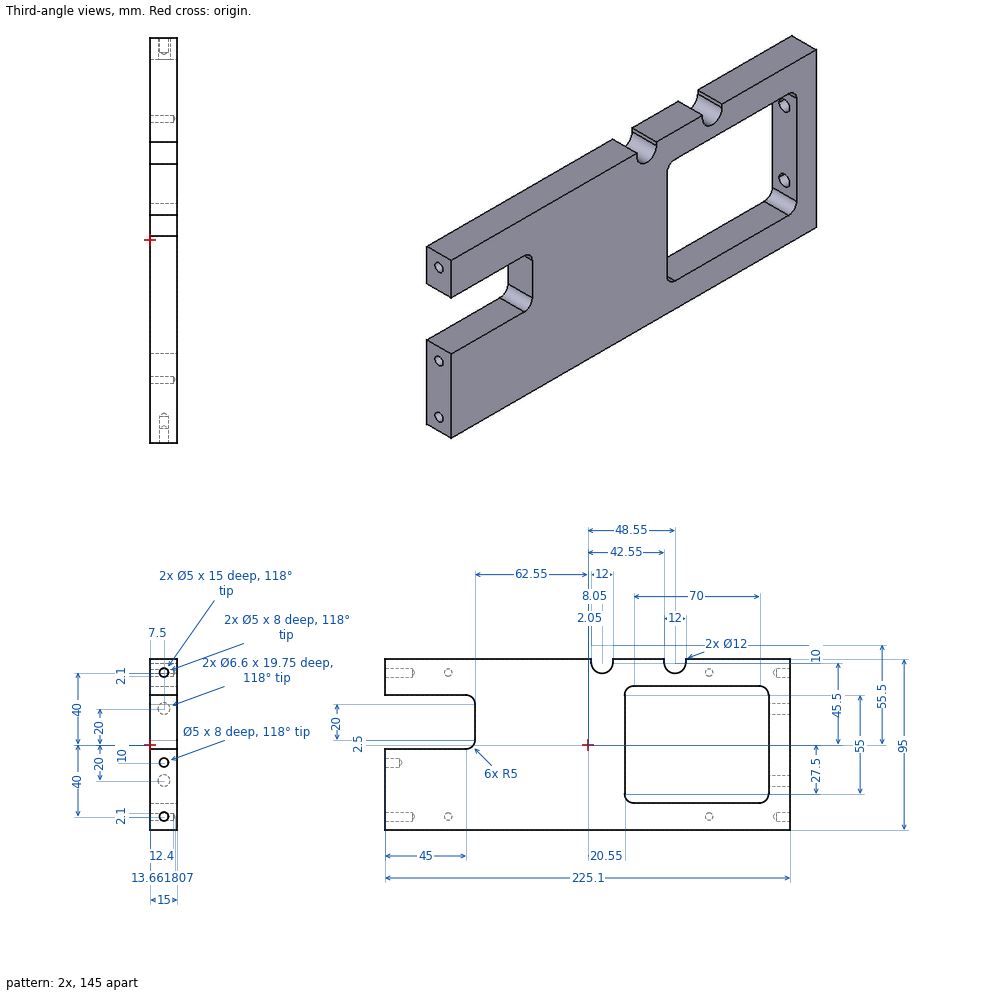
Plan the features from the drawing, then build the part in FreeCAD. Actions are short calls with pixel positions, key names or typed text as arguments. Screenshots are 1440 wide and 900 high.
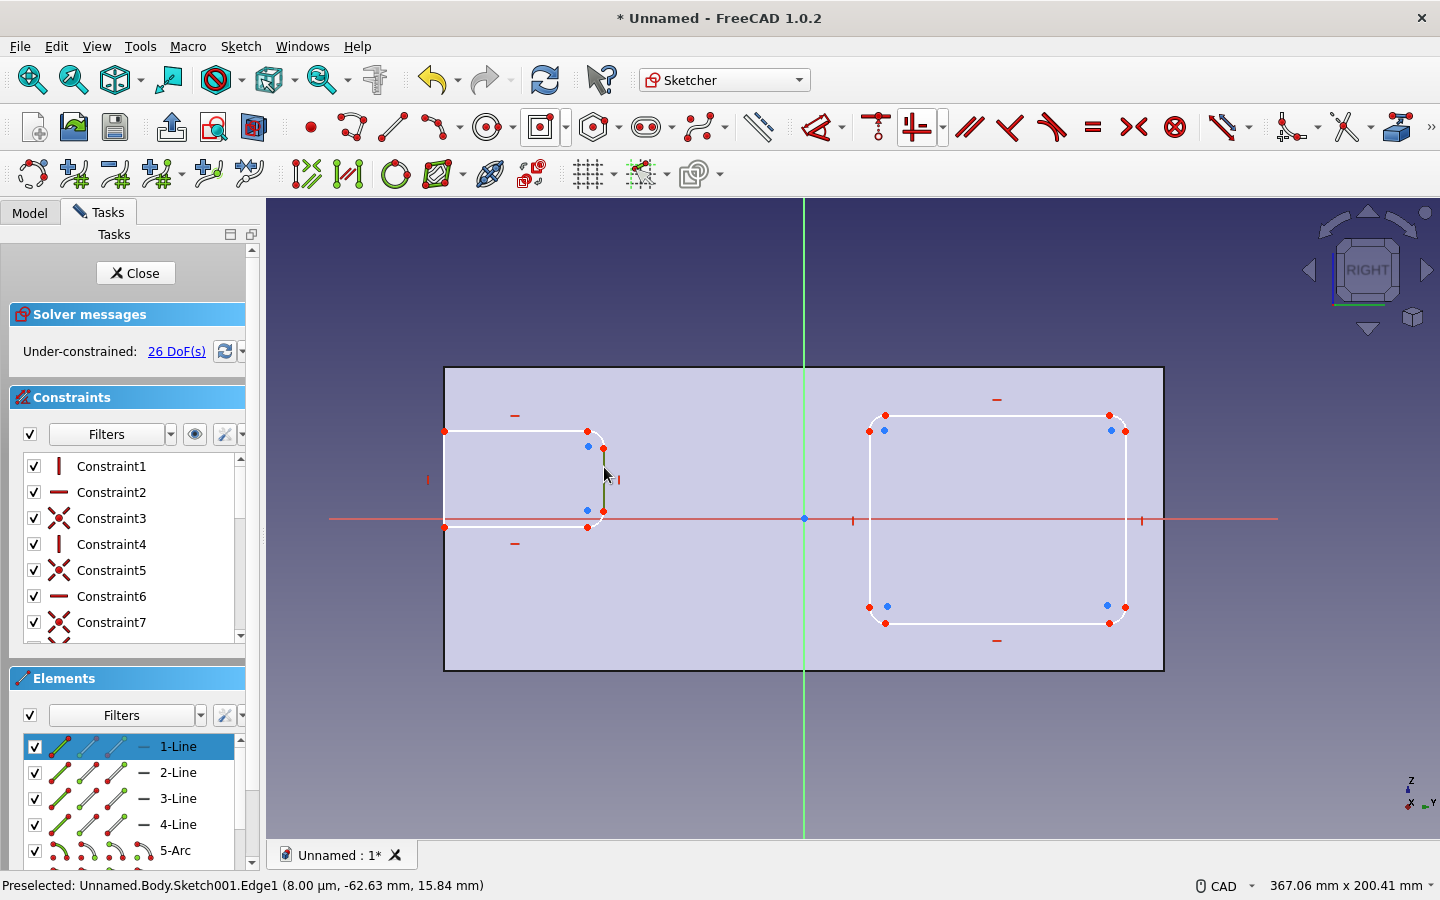
click(599, 522)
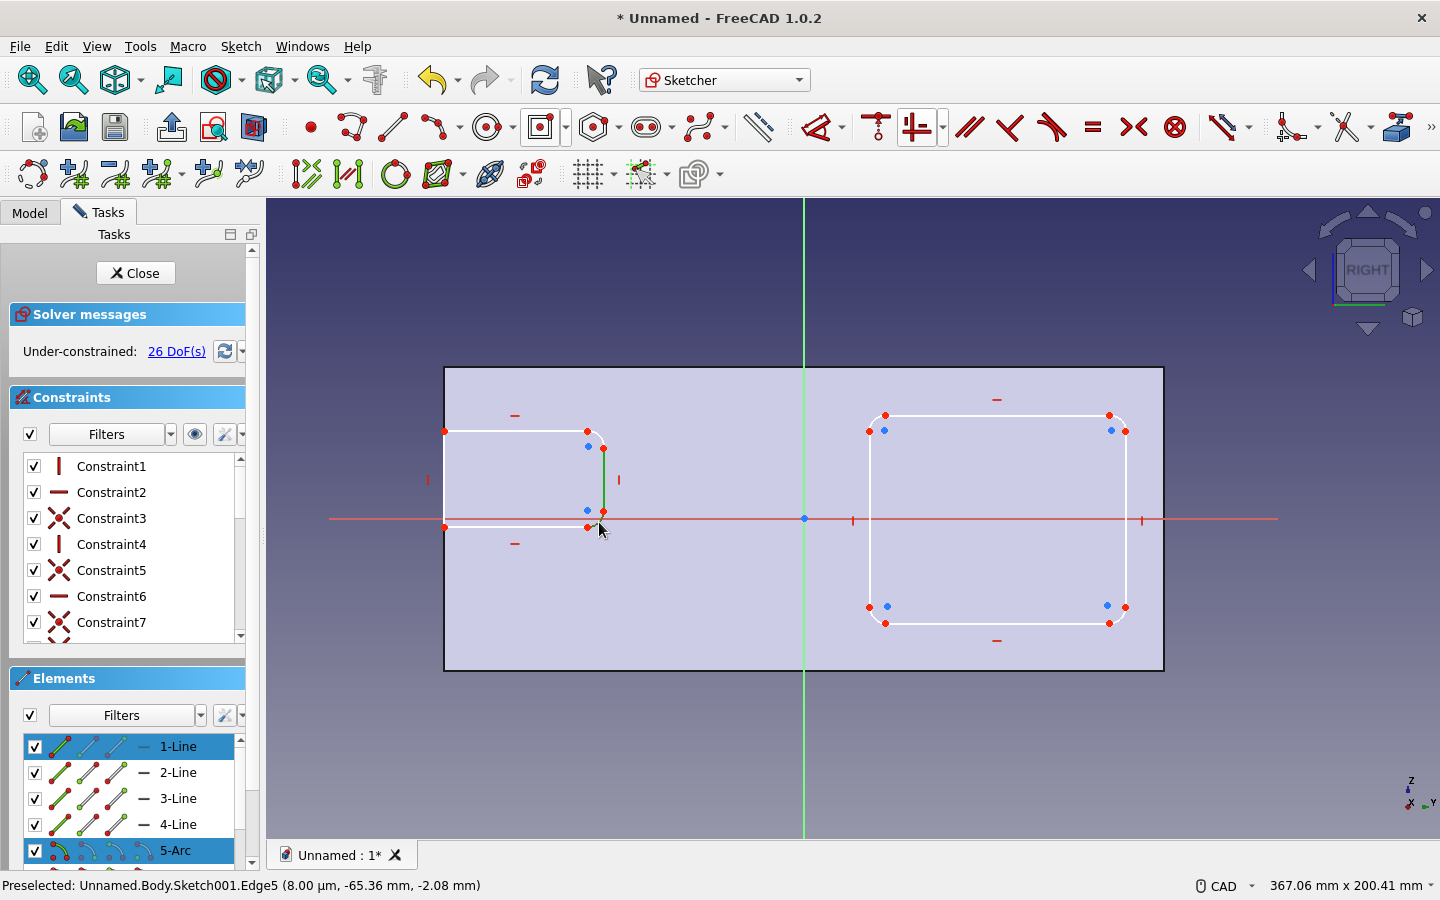
click(1052, 128)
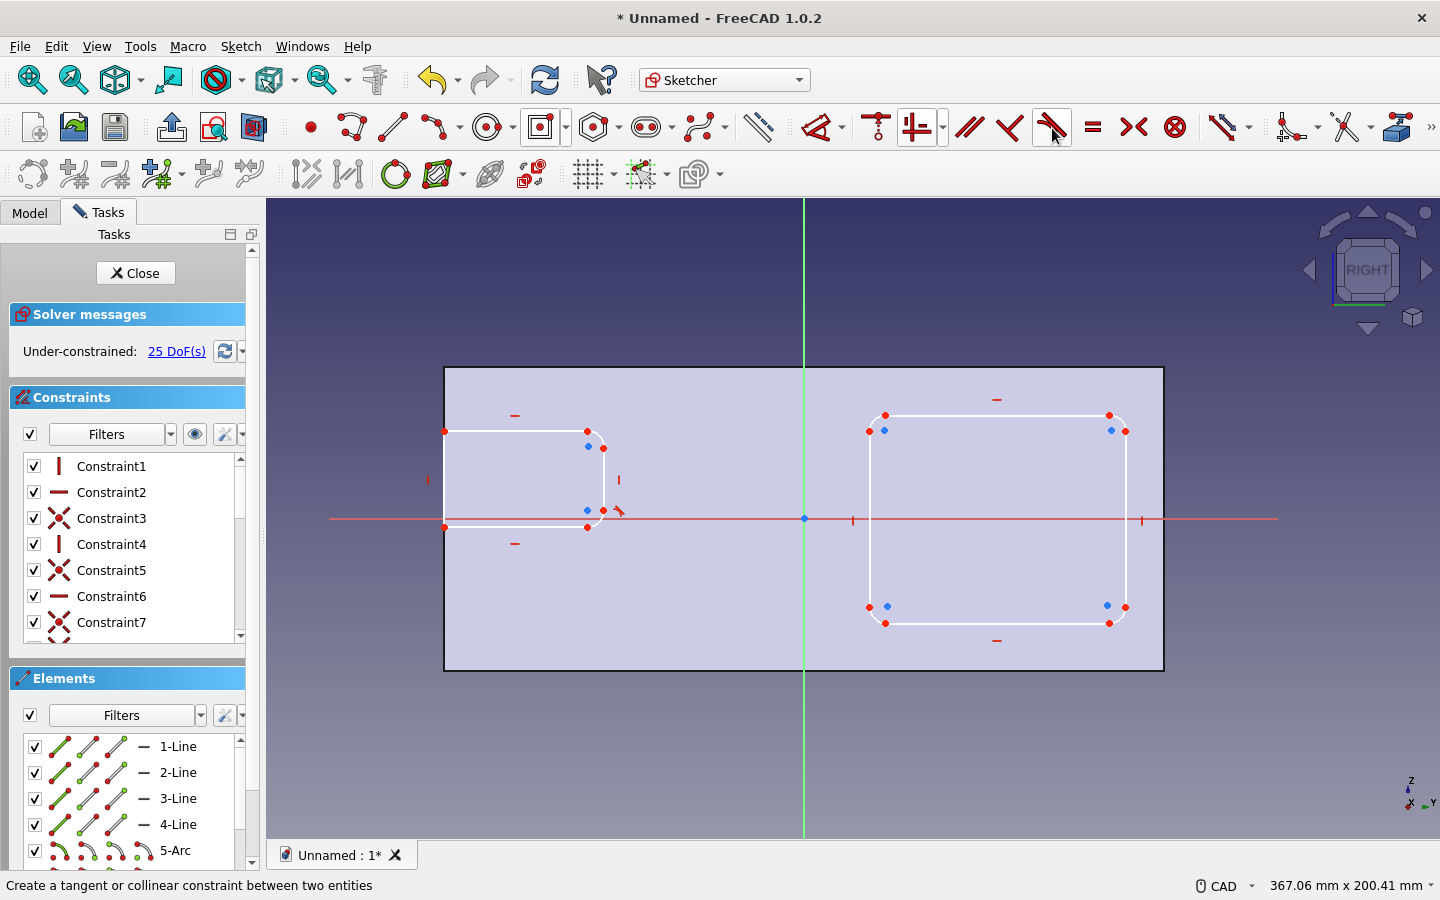
click(604, 467)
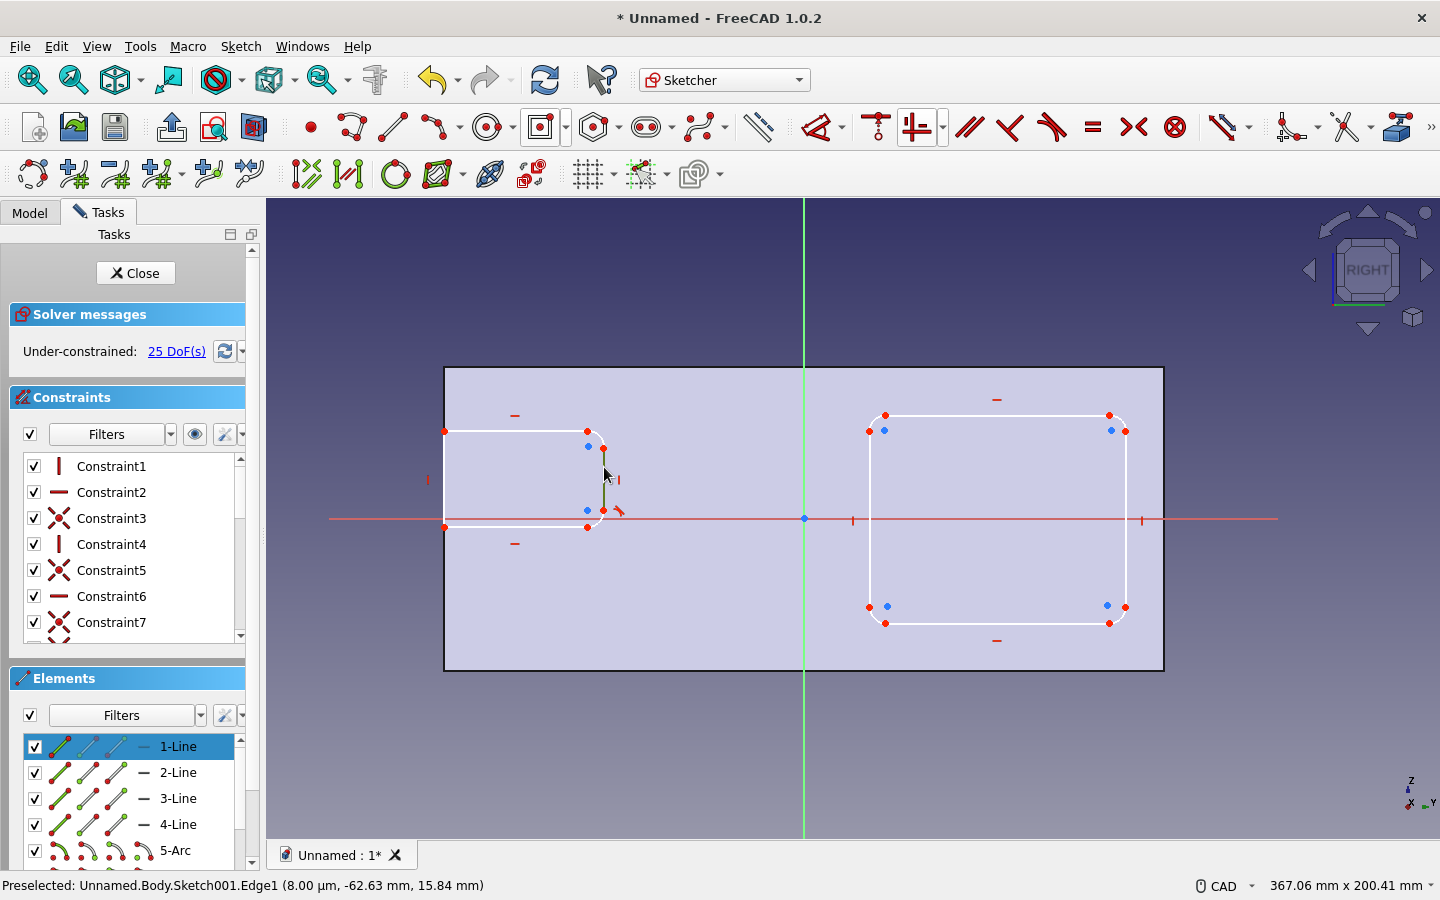
click(600, 436)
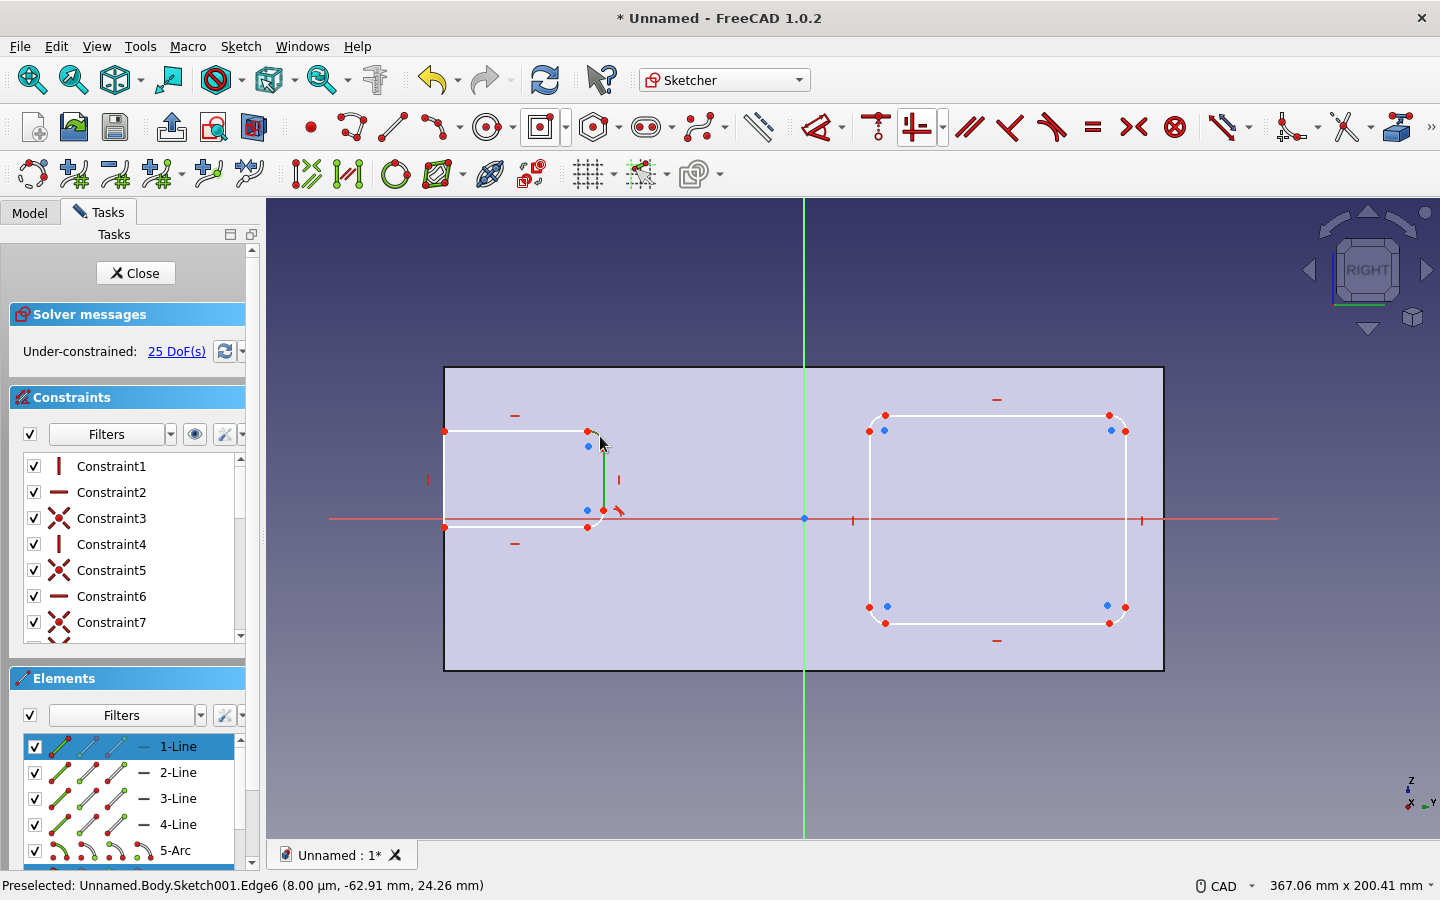
click(1052, 128)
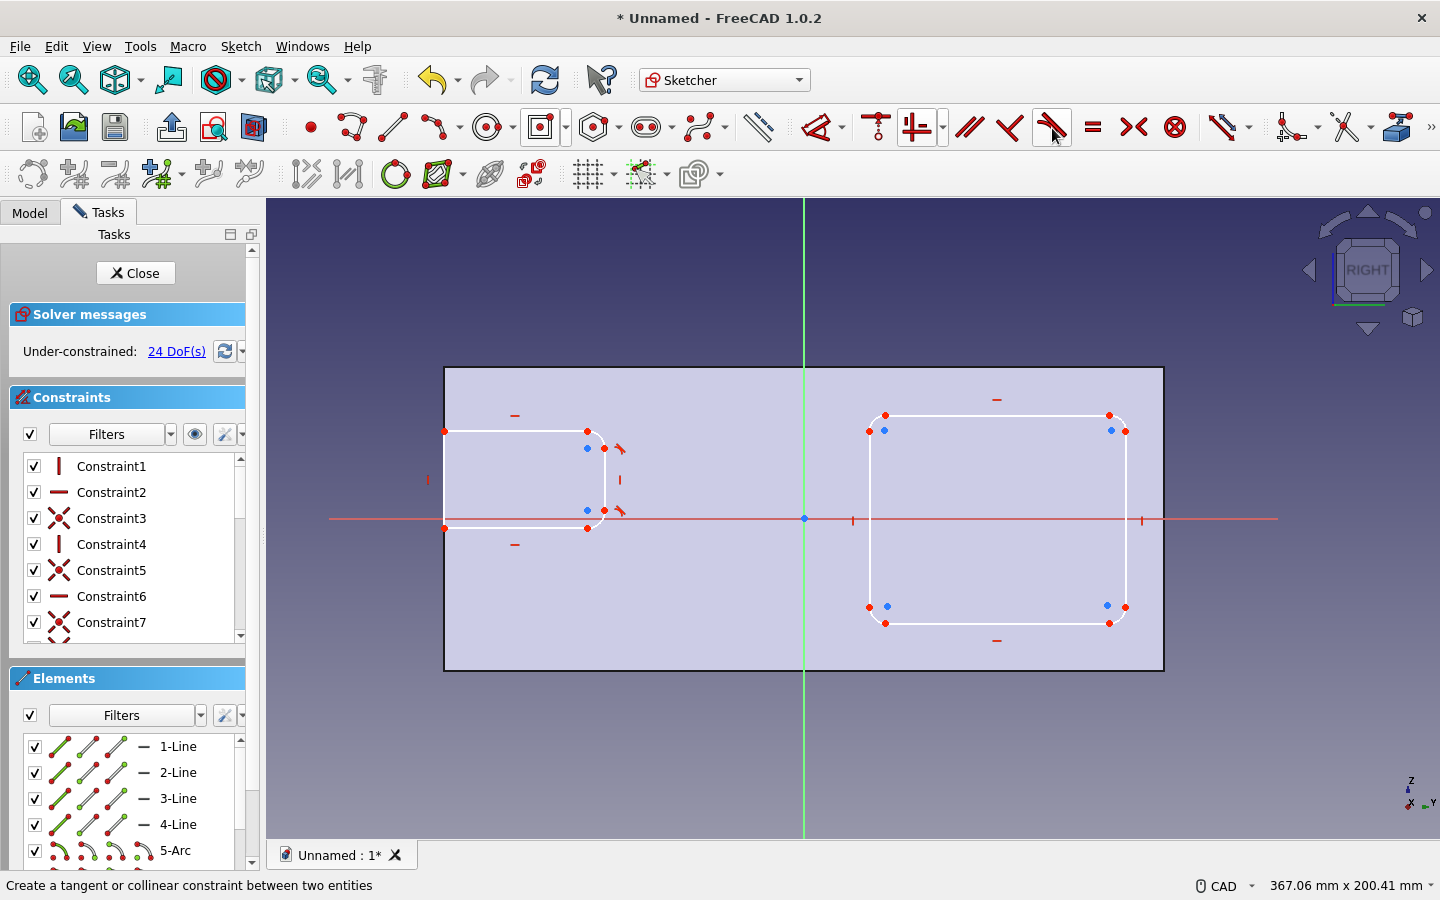
scroll(545, 528, up, 2)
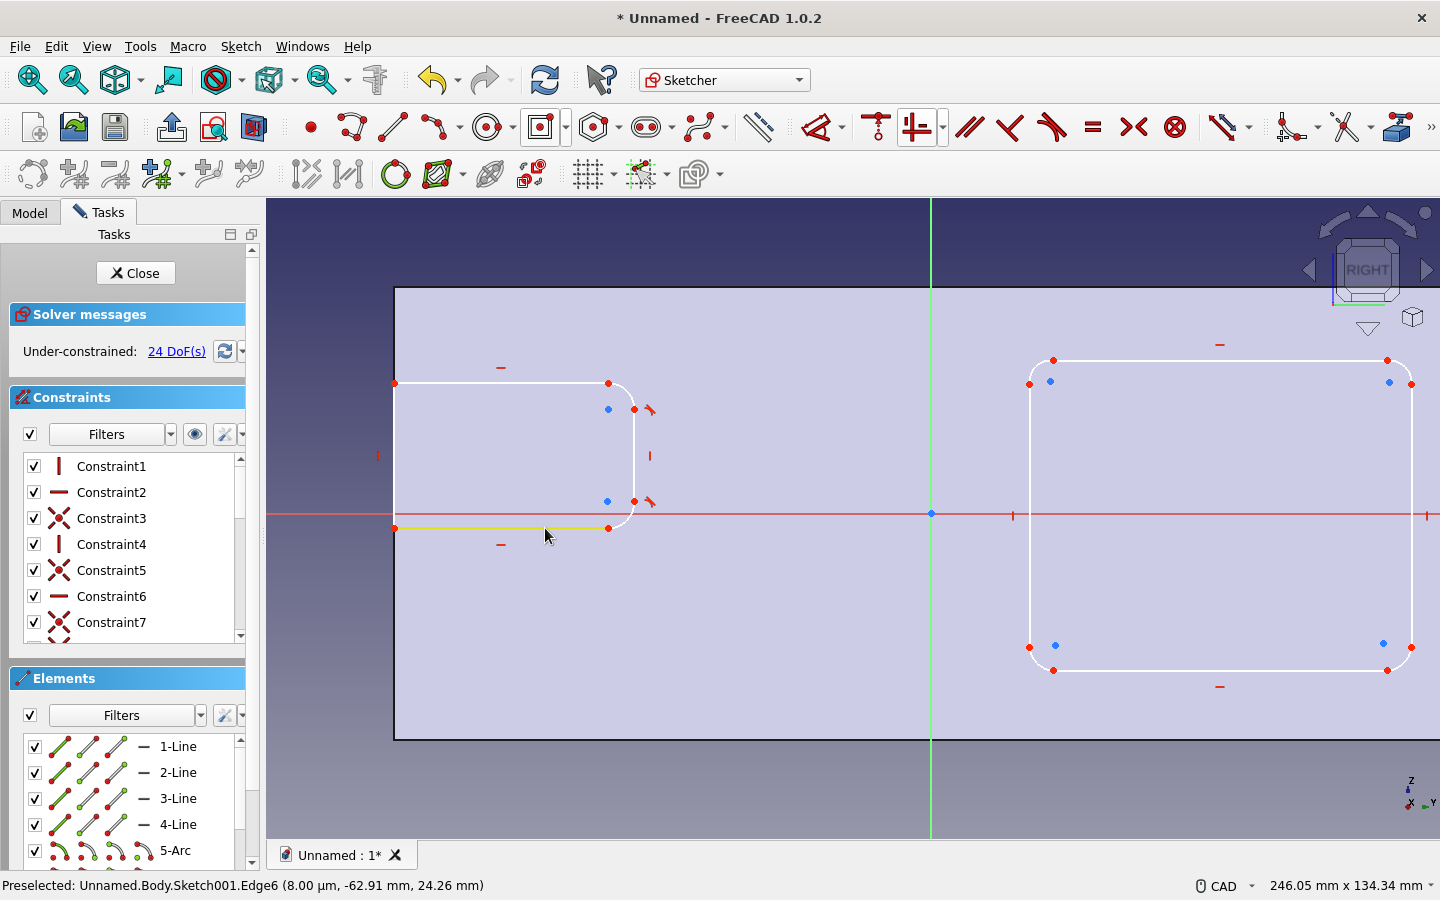
click(544, 528)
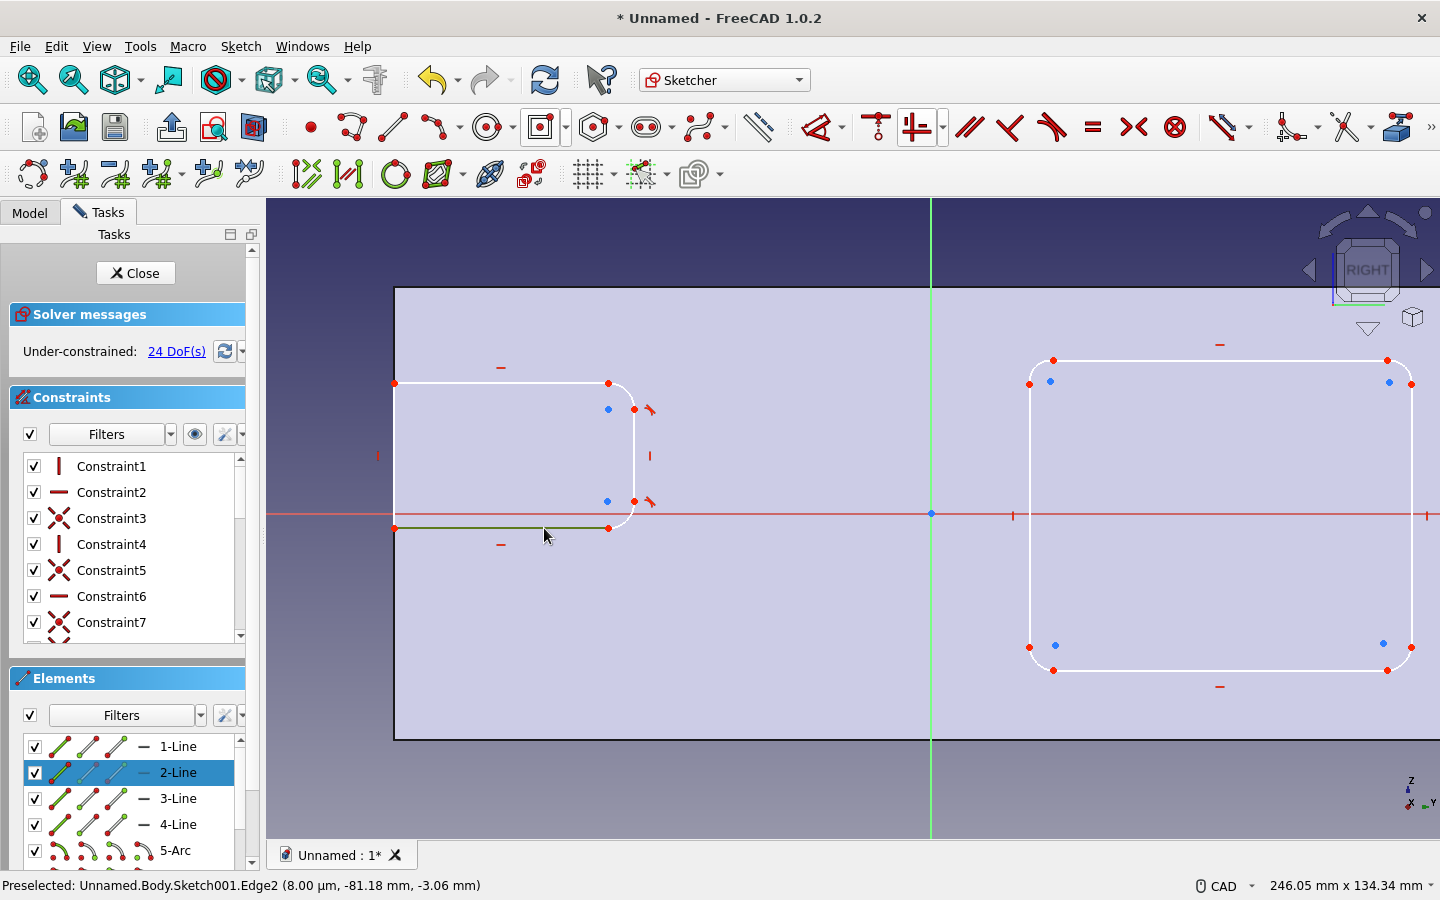
click(620, 525)